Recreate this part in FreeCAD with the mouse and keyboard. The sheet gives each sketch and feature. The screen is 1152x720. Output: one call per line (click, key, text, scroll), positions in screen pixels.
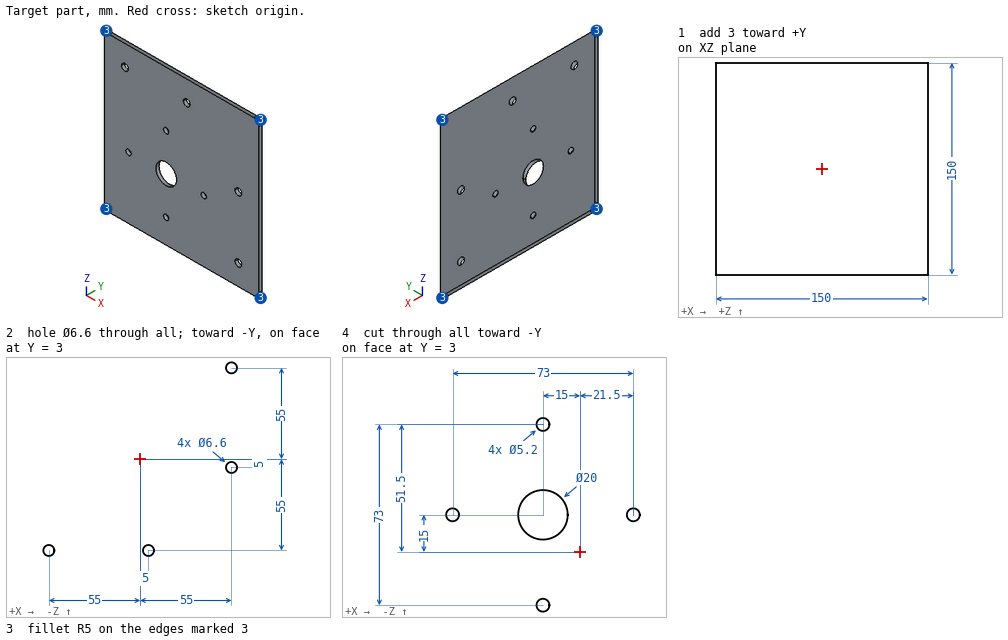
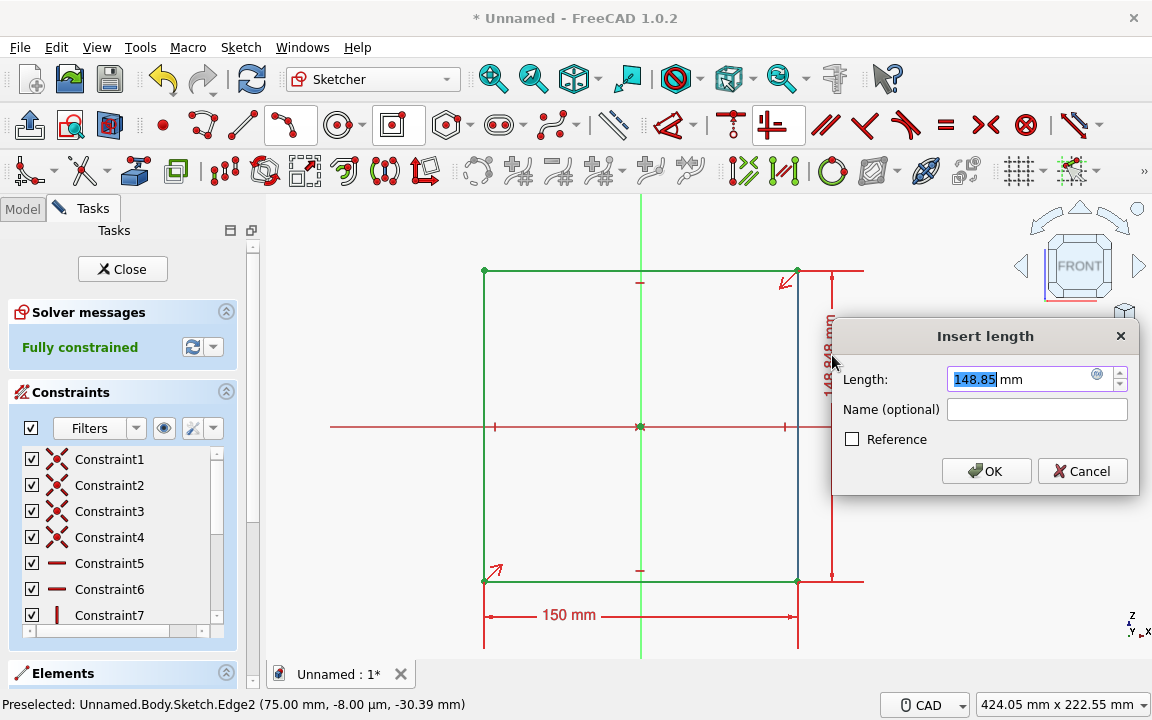
text(150)
key(Return)
key(Escape)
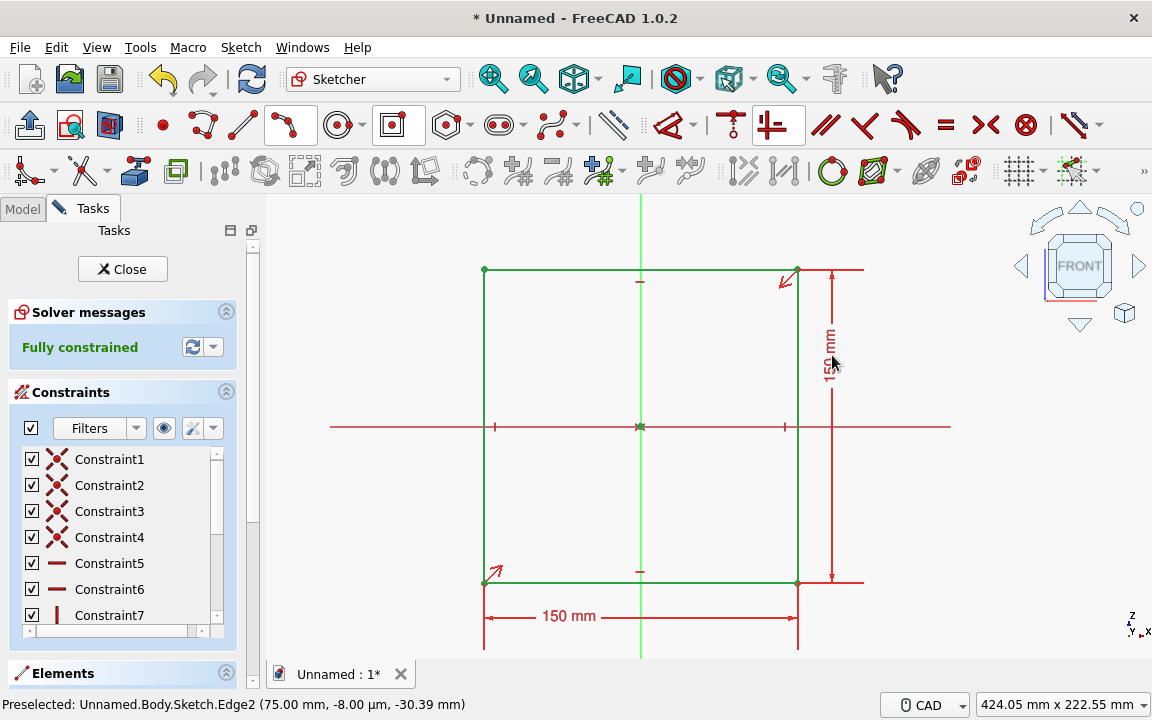
click(123, 269)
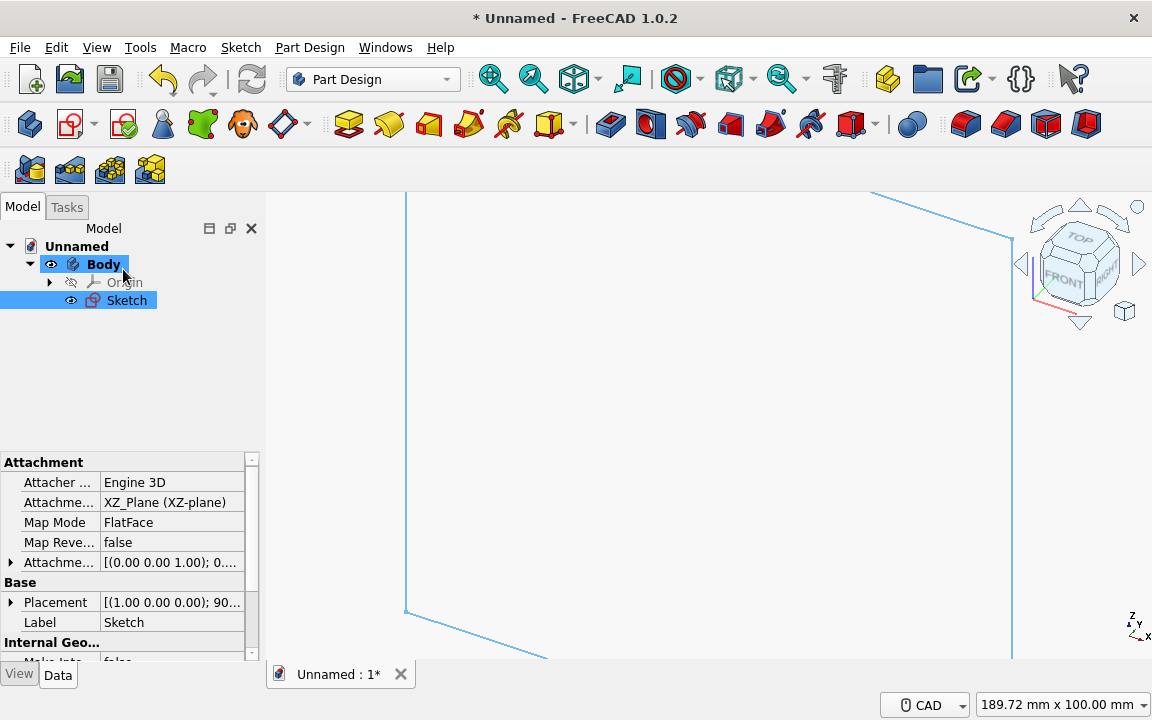
click(350, 124)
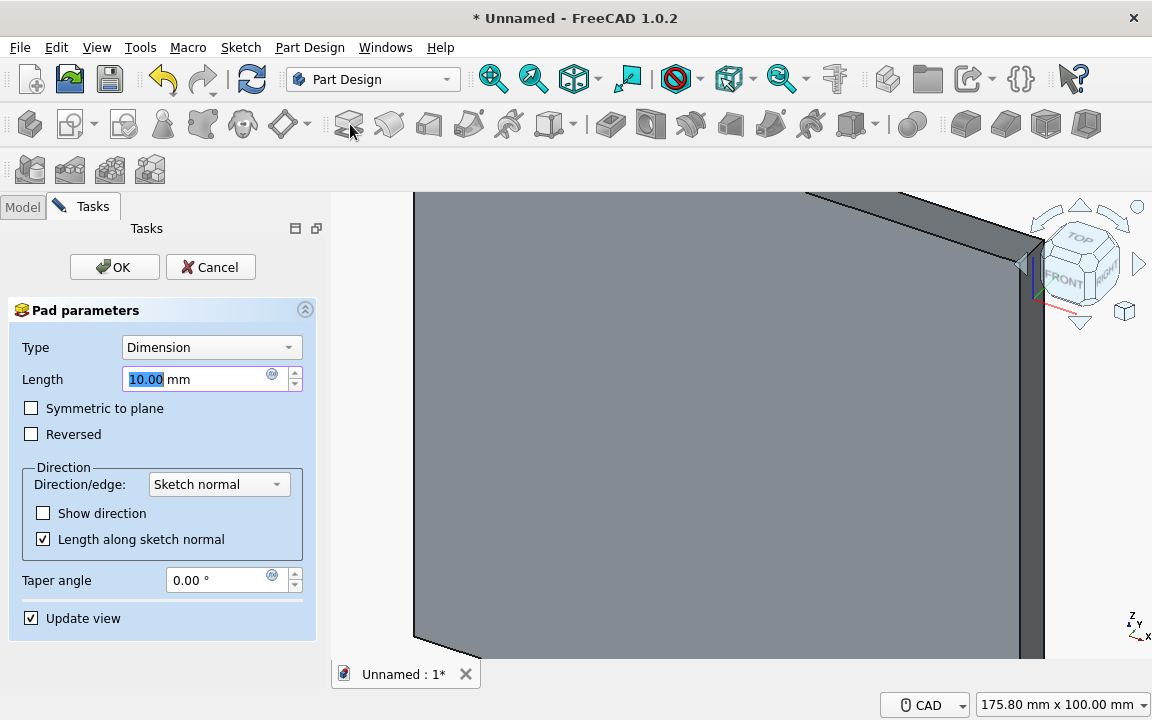
text(3)
key(Tab)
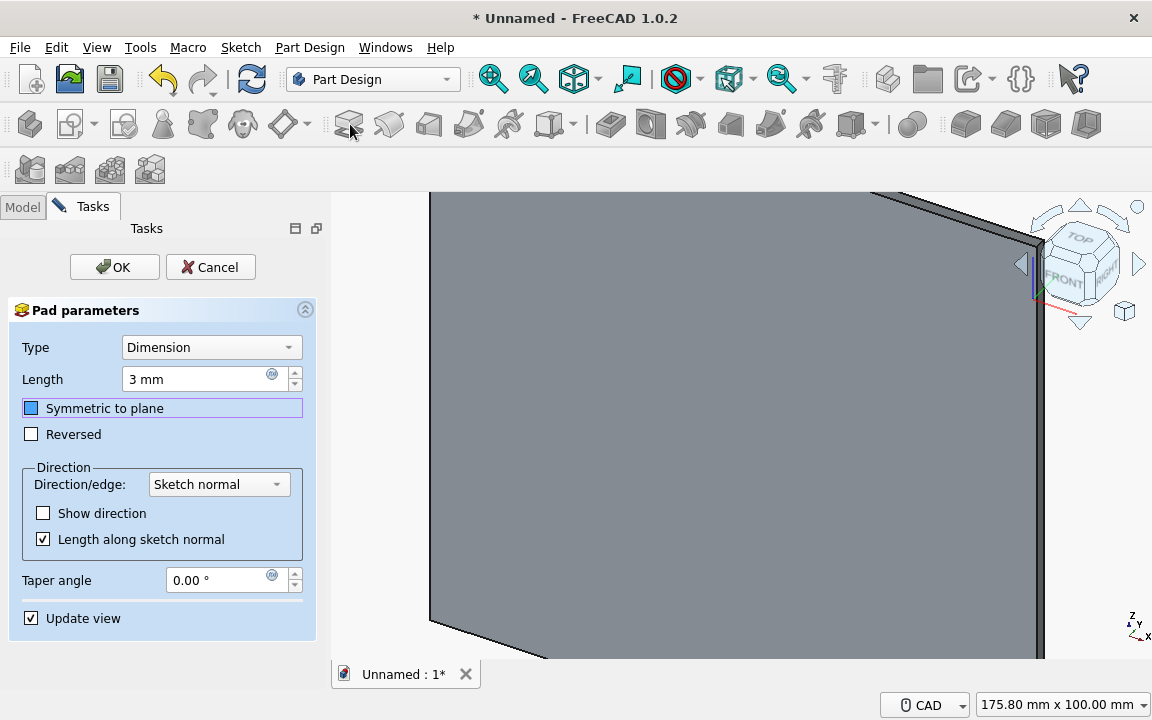
click(30, 434)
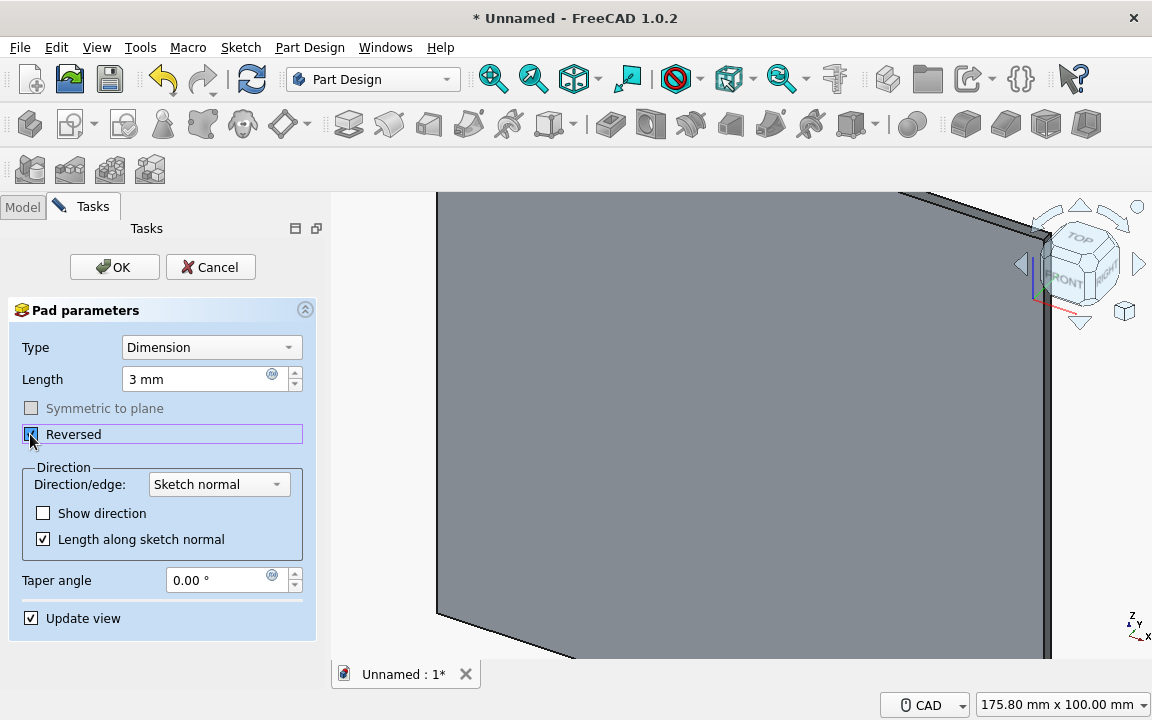
click(115, 267)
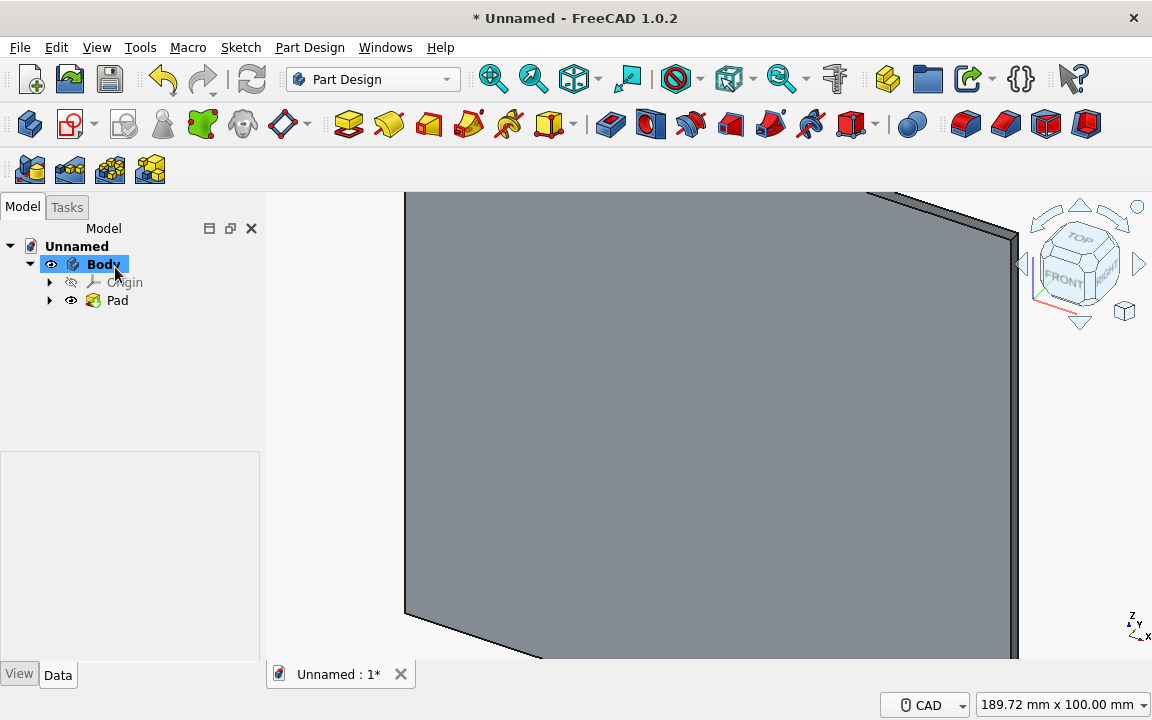
click(494, 80)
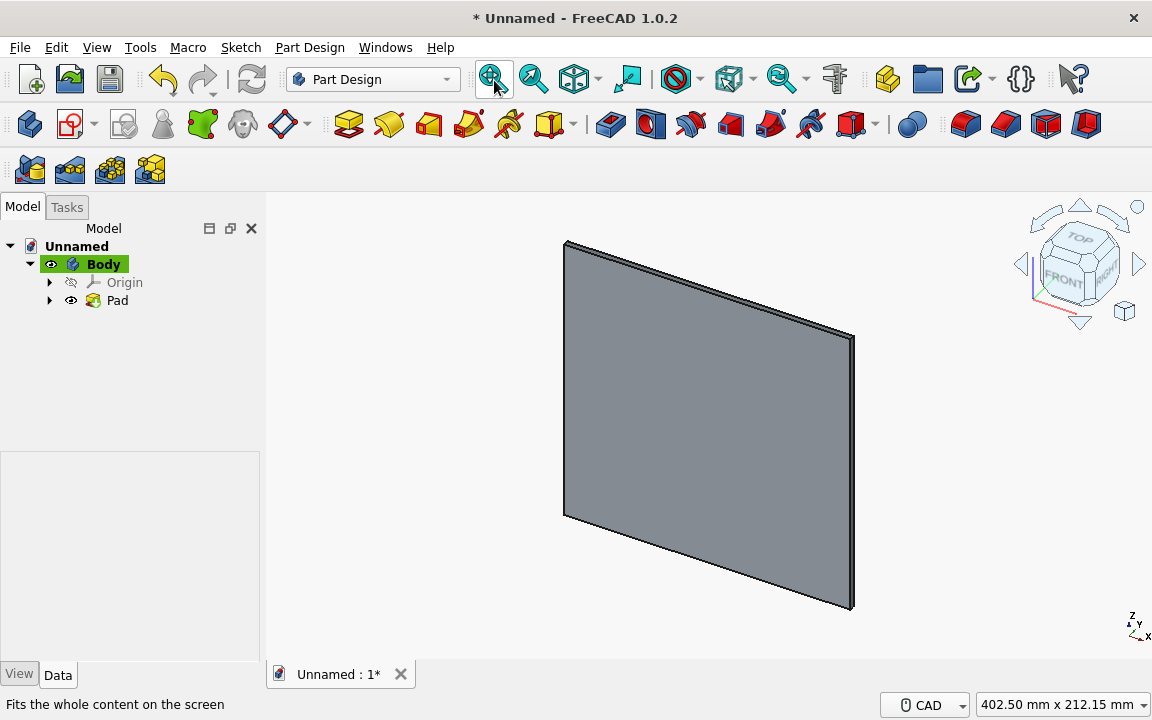
key(4)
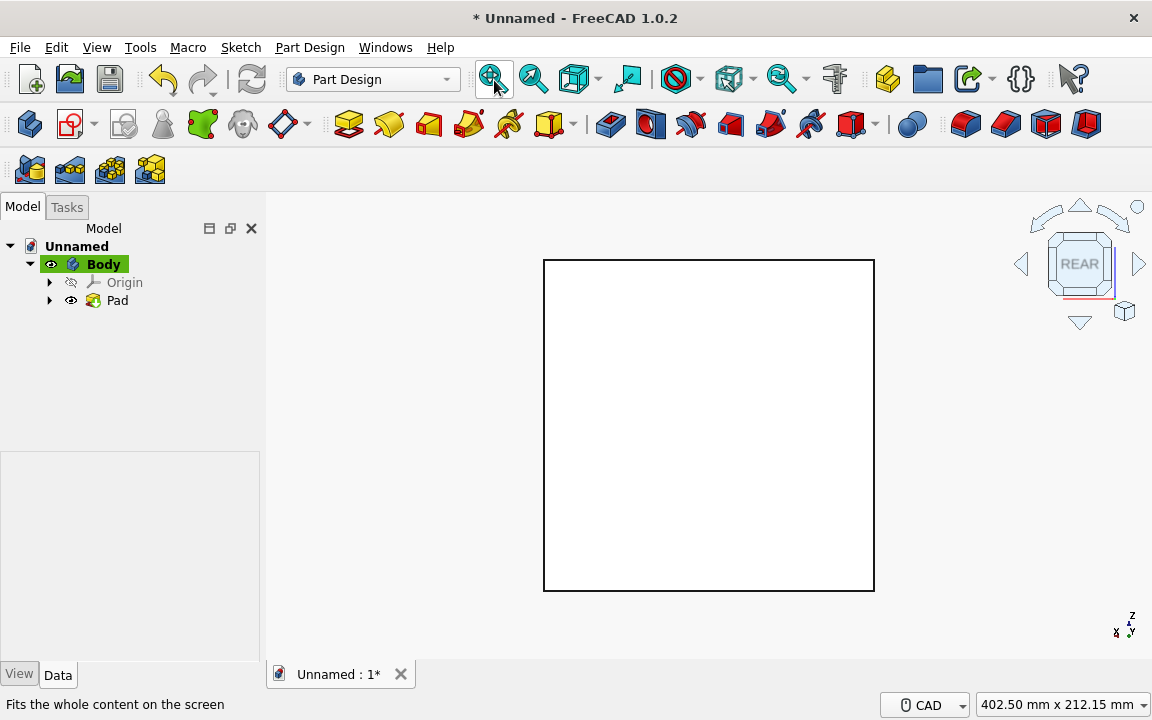
click(709, 425)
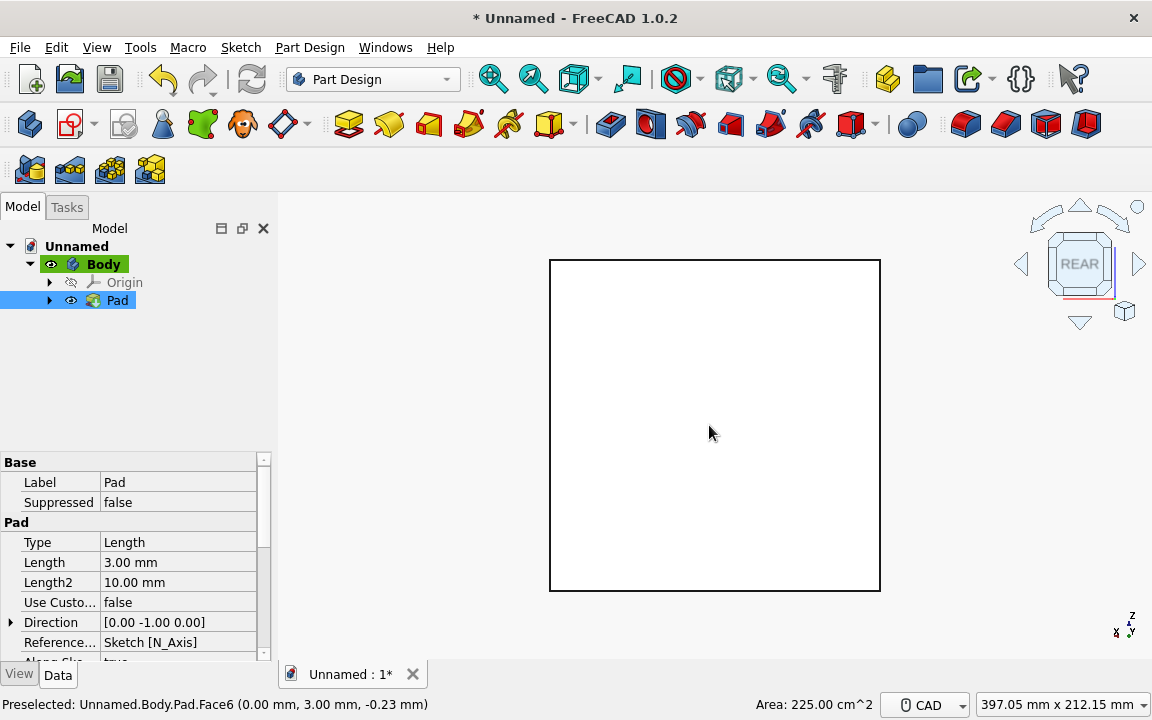
click(70, 124)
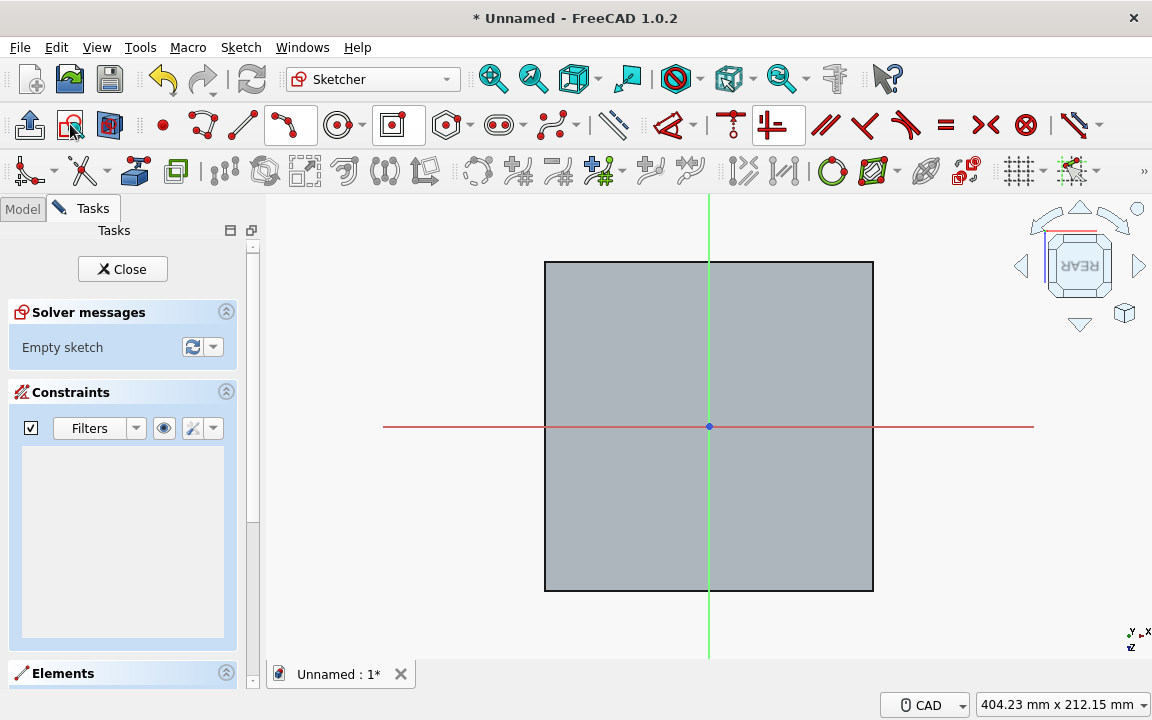
click(338, 126)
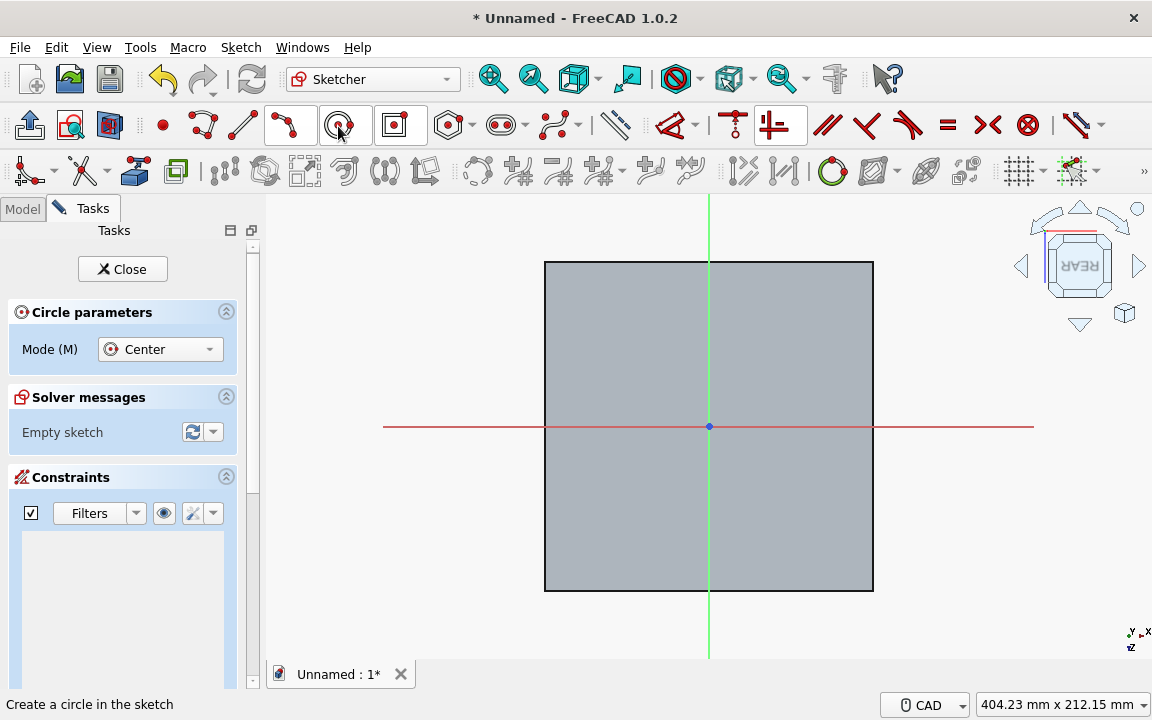
scroll(830, 437, up, 6)